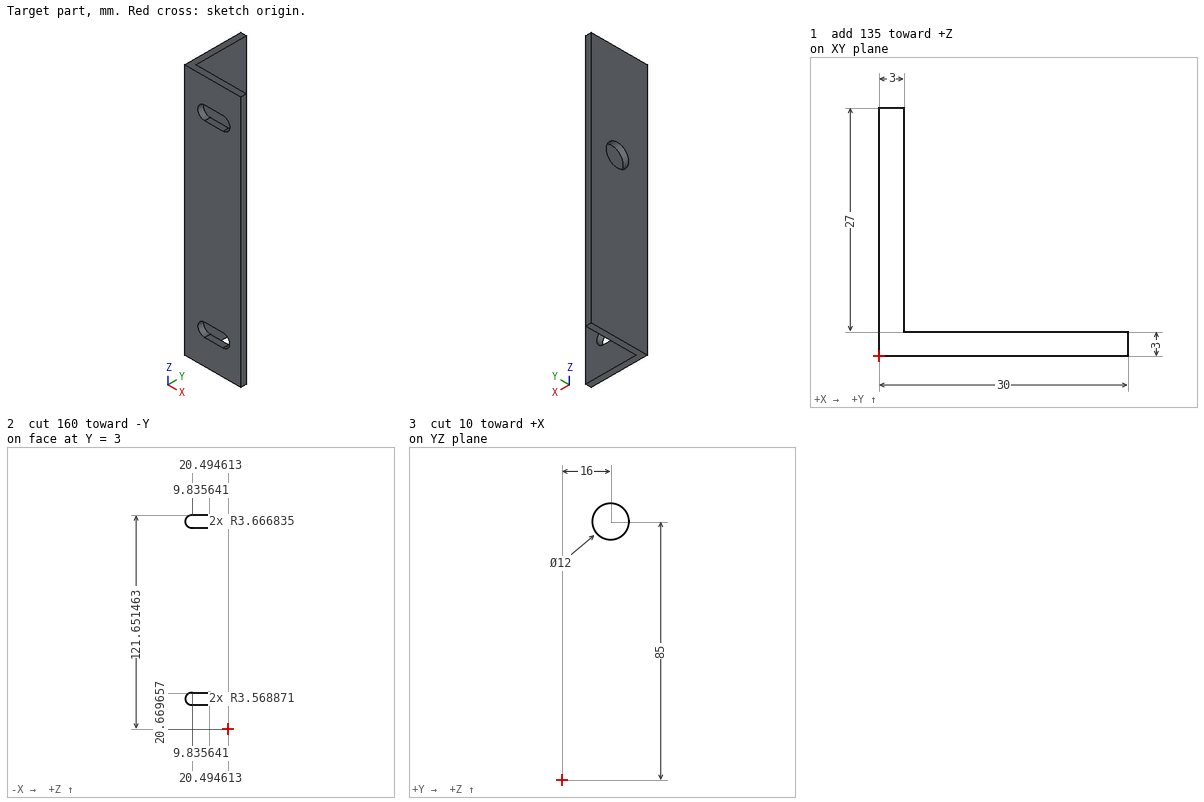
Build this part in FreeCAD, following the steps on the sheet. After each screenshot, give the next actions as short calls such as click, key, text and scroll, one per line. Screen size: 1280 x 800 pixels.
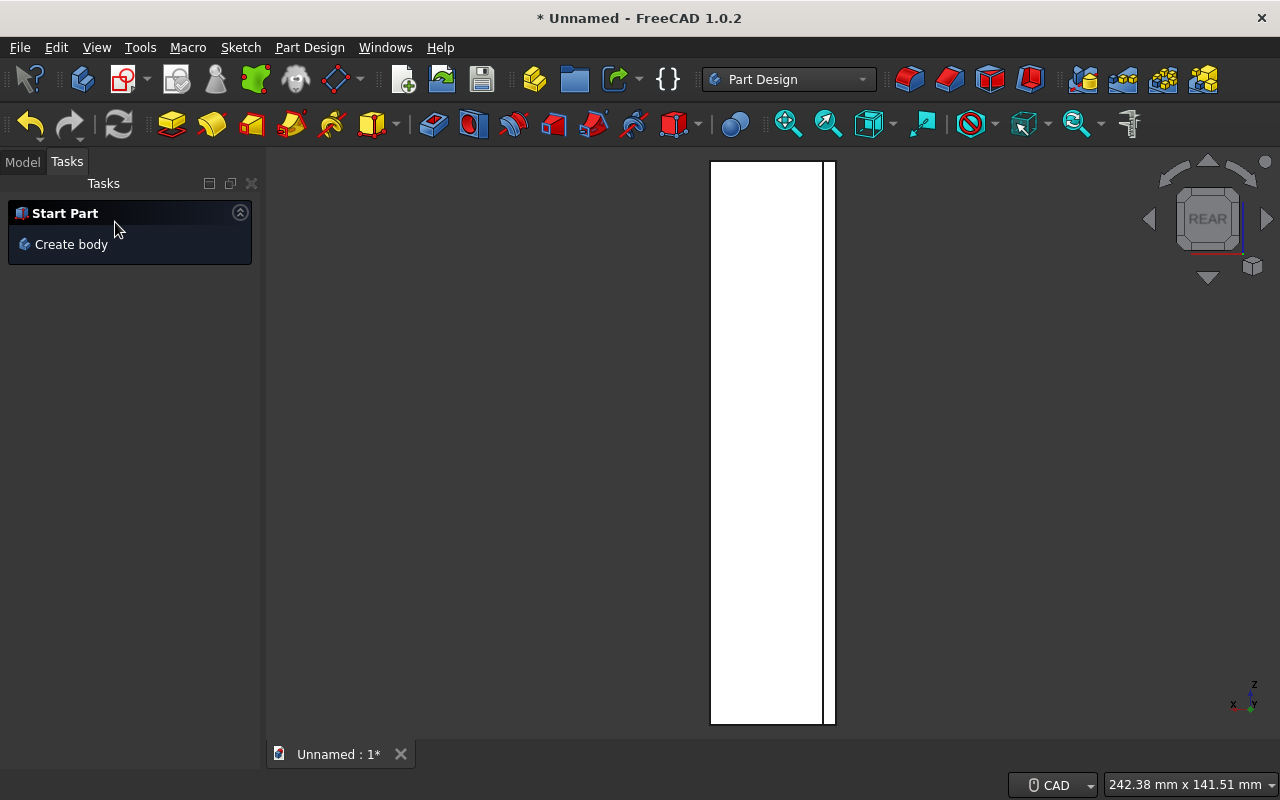
click(767, 281)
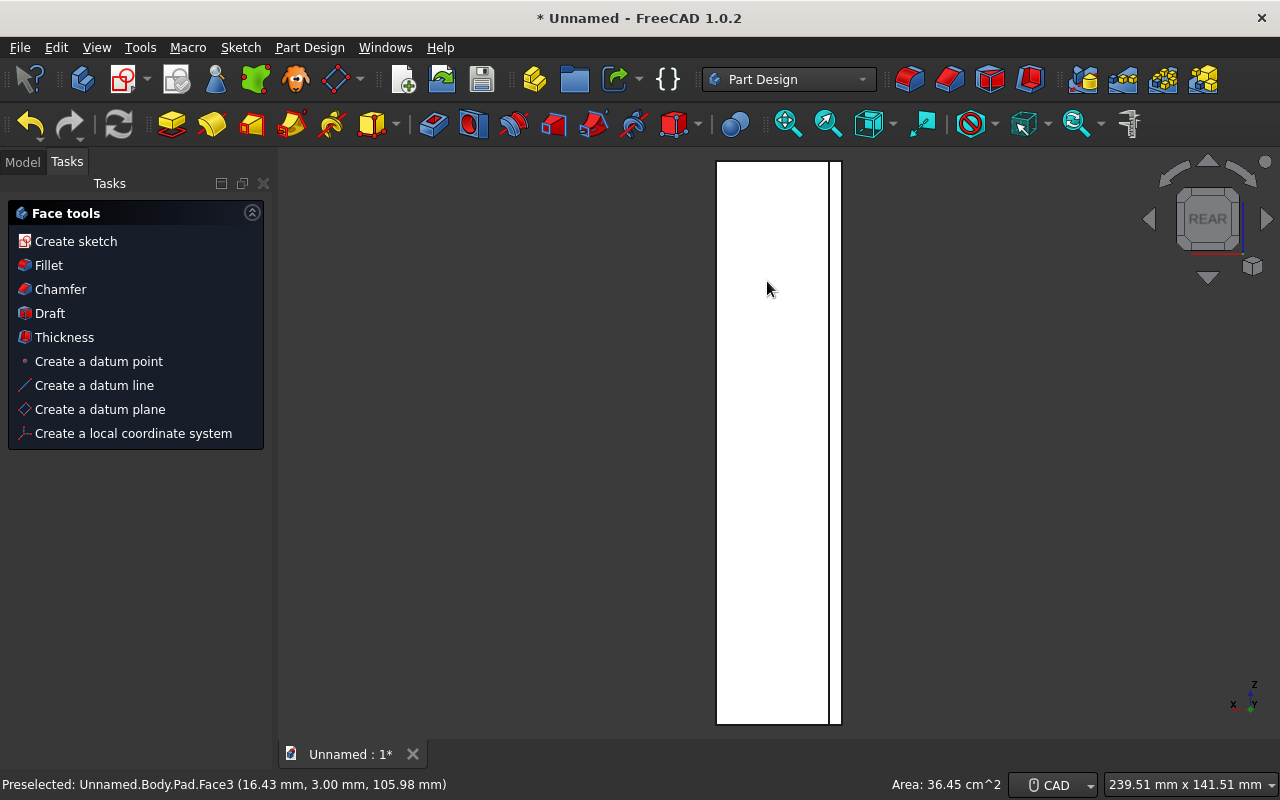
click(124, 80)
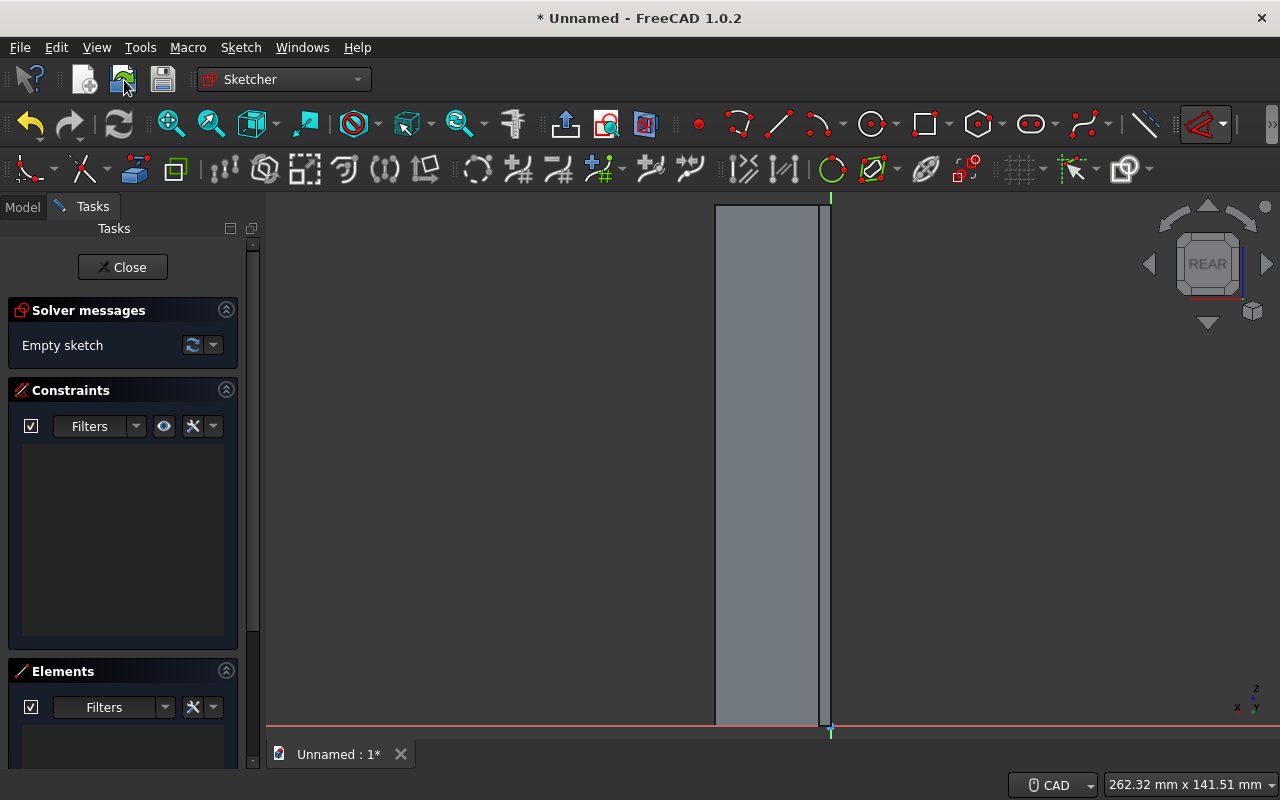
key(q)
key(s)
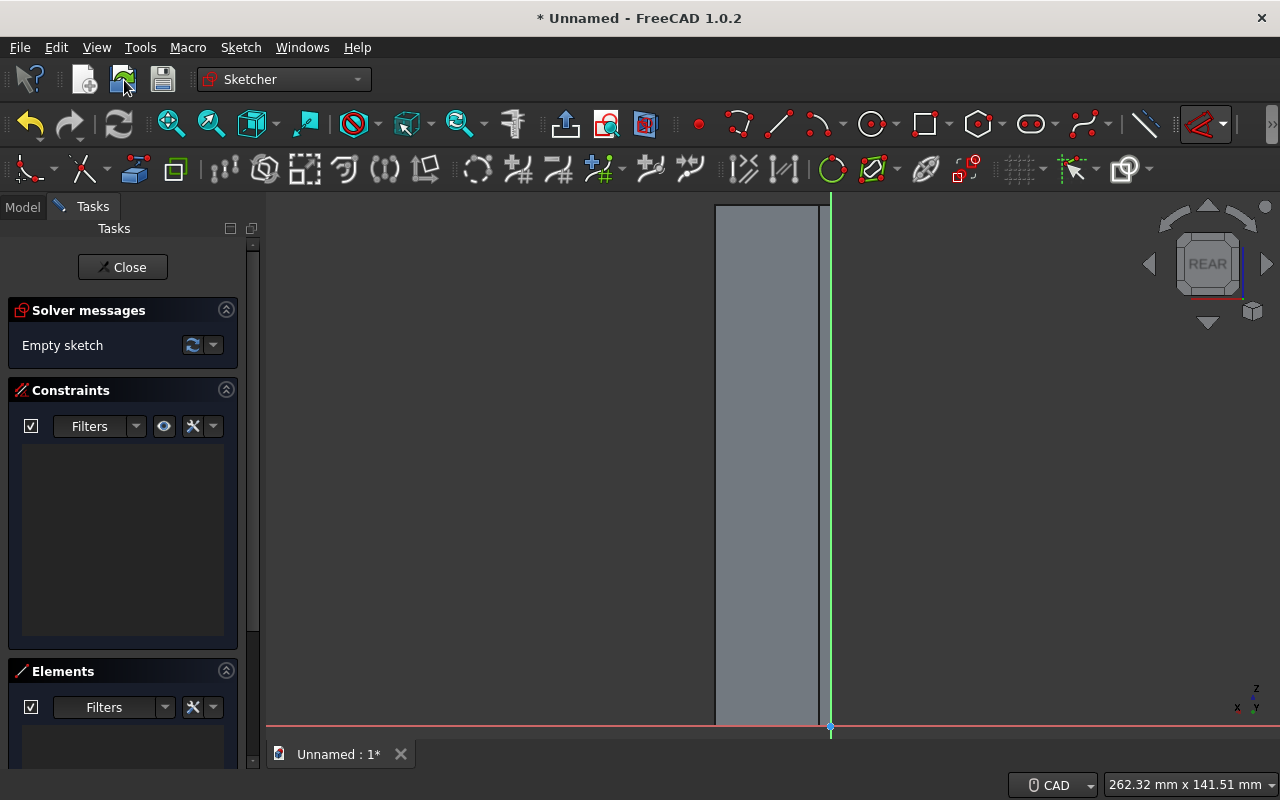
scroll(542, 413, down, 2)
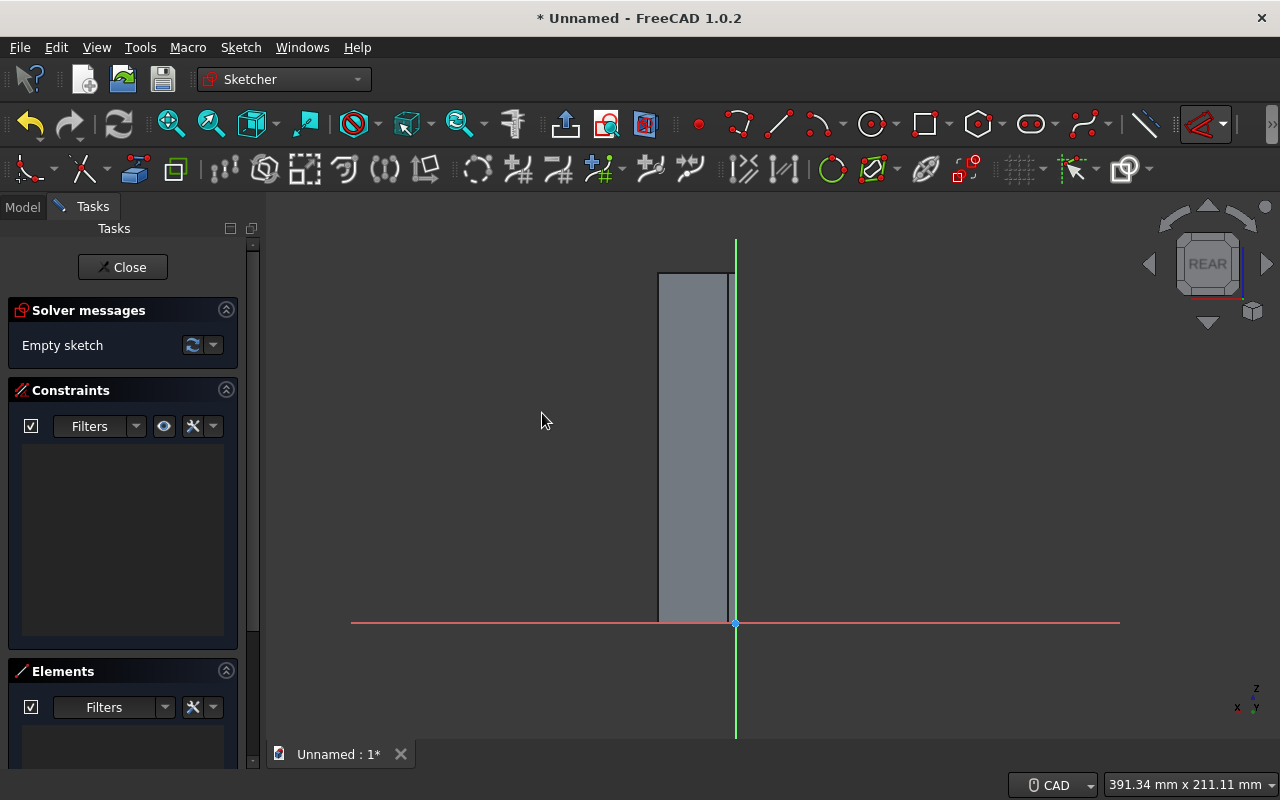
click(1032, 124)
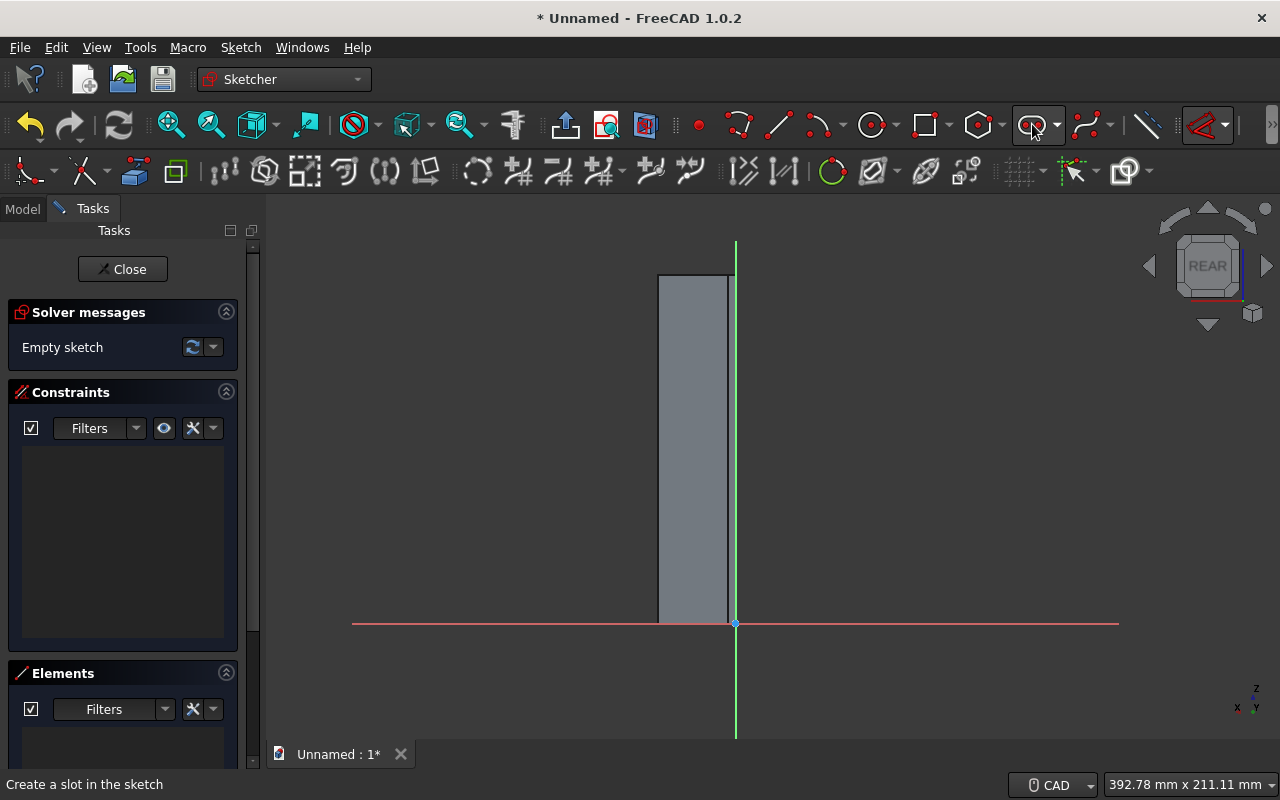
scroll(683, 579, up, 5)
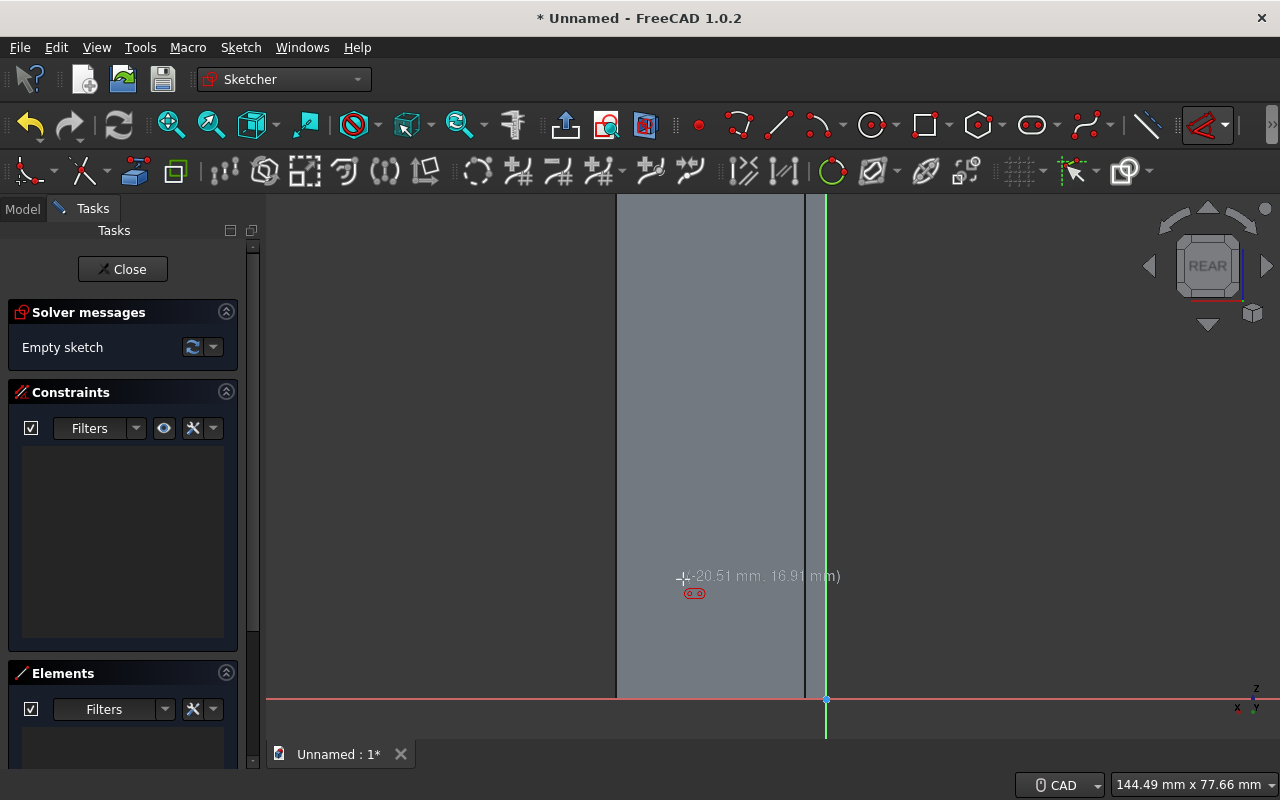
click(682, 579)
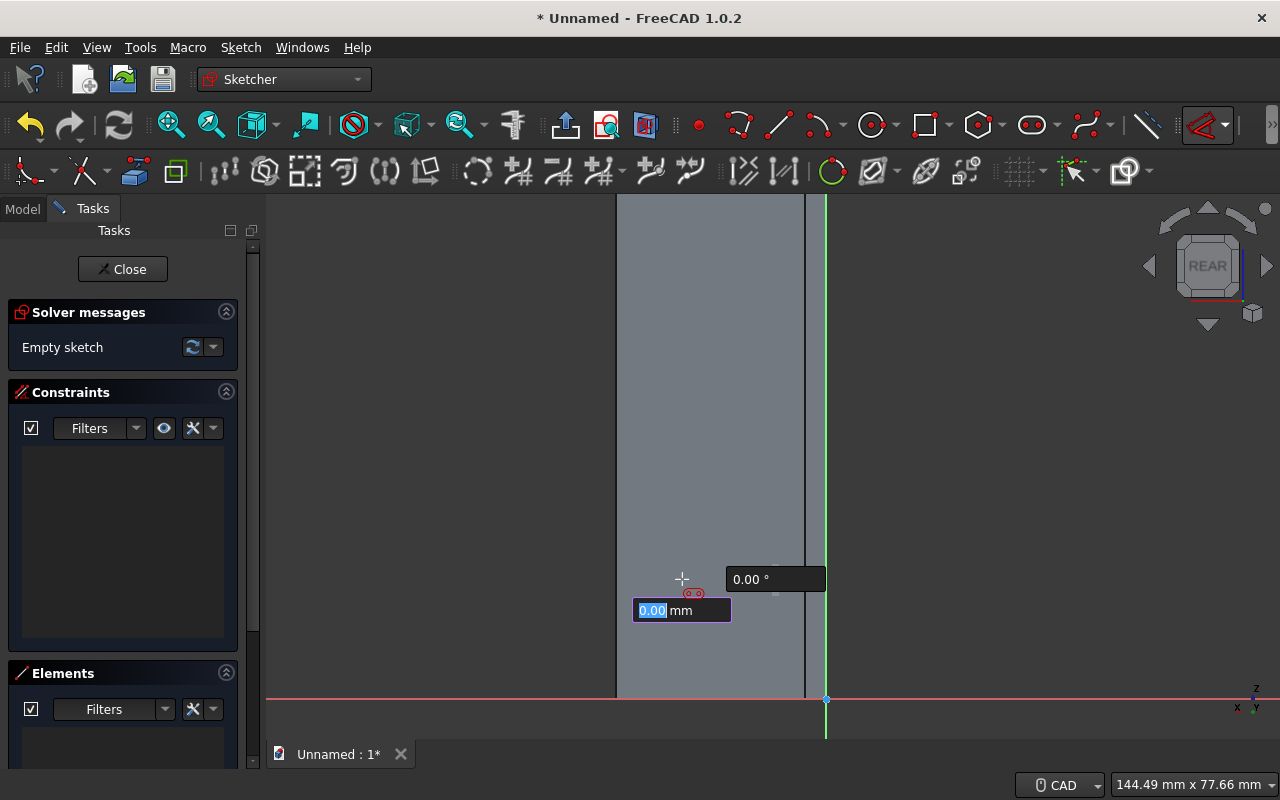
click(751, 579)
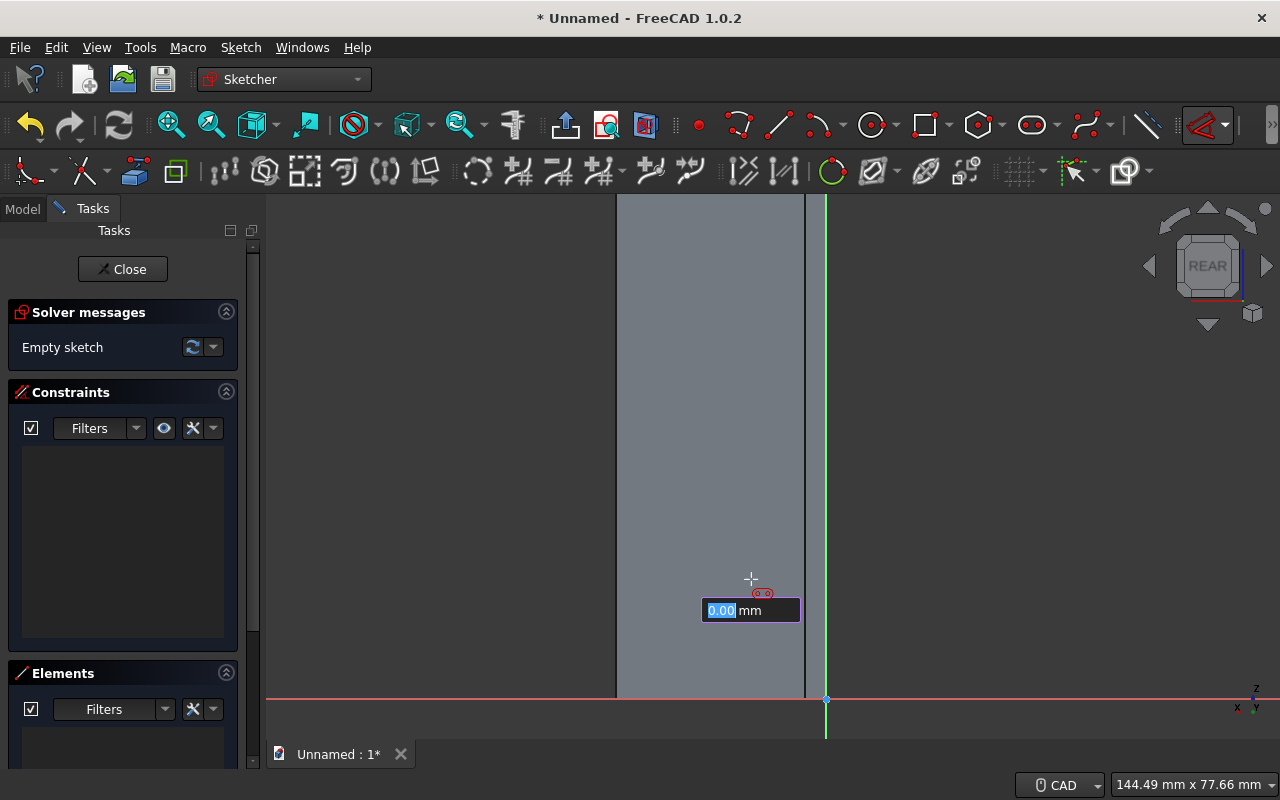
click(717, 604)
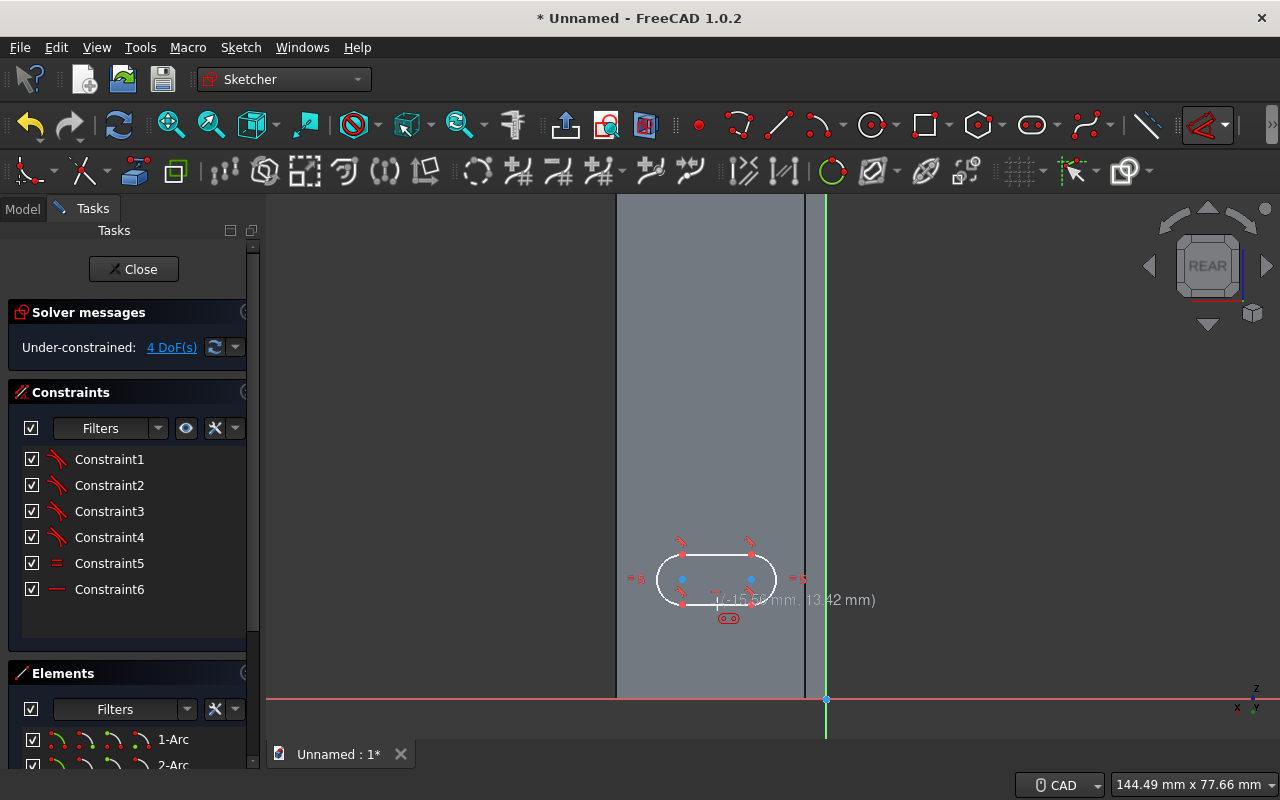
scroll(683, 580, down, 5)